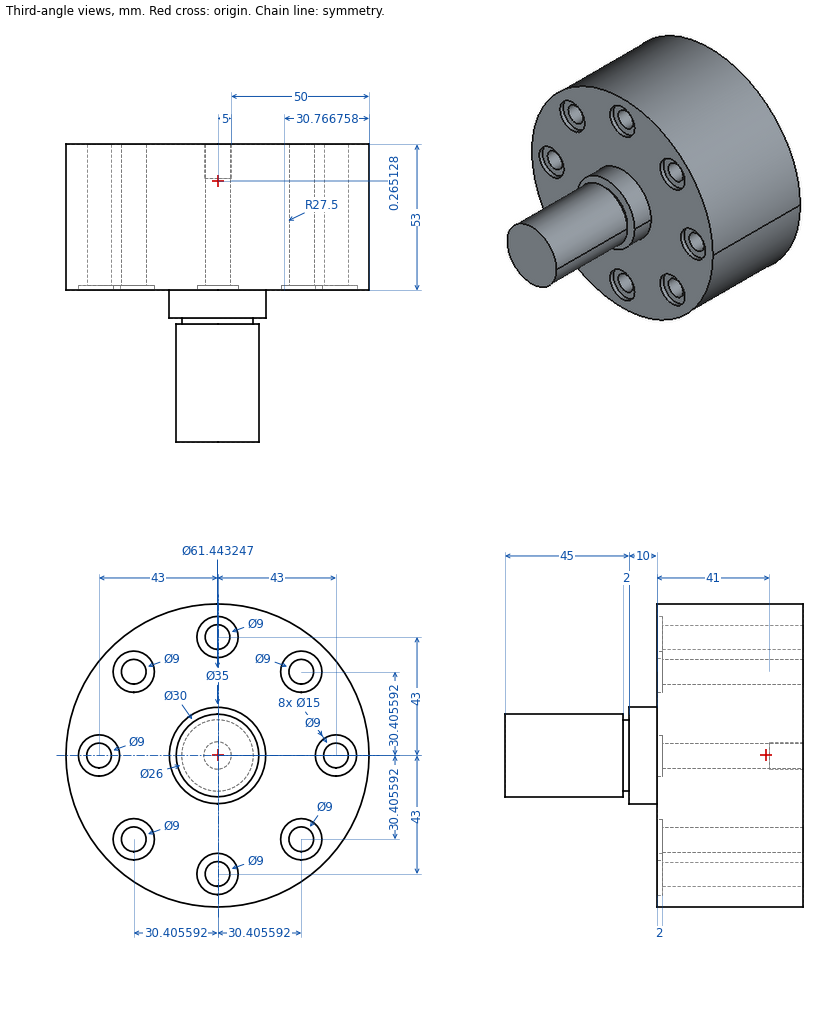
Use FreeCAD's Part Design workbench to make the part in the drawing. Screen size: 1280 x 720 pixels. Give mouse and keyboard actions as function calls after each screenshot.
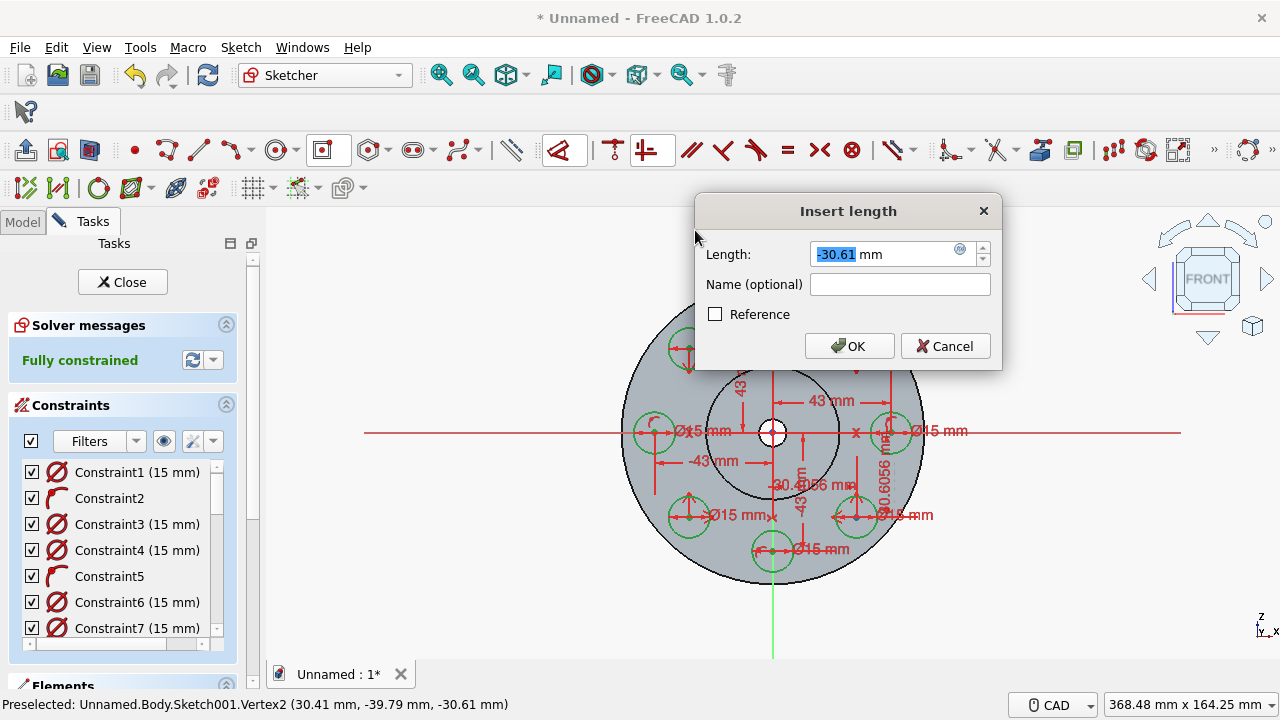
text(-30.405592)
key(Return)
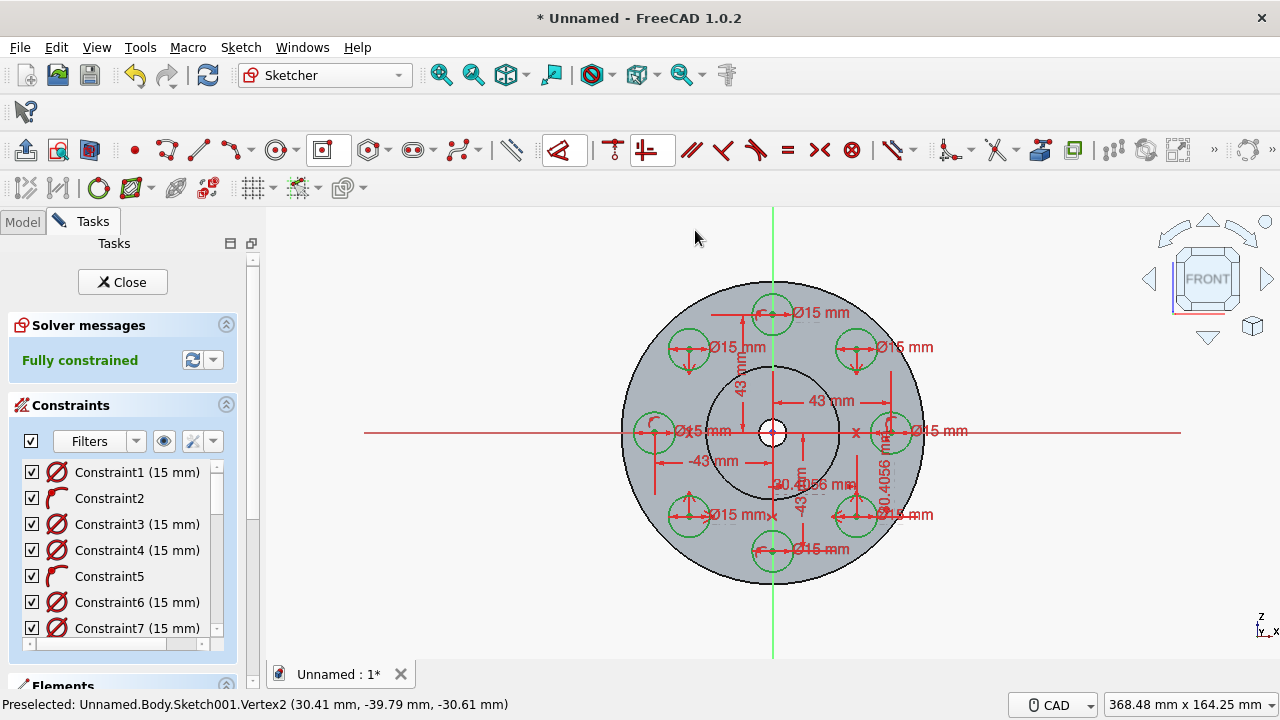
click(123, 282)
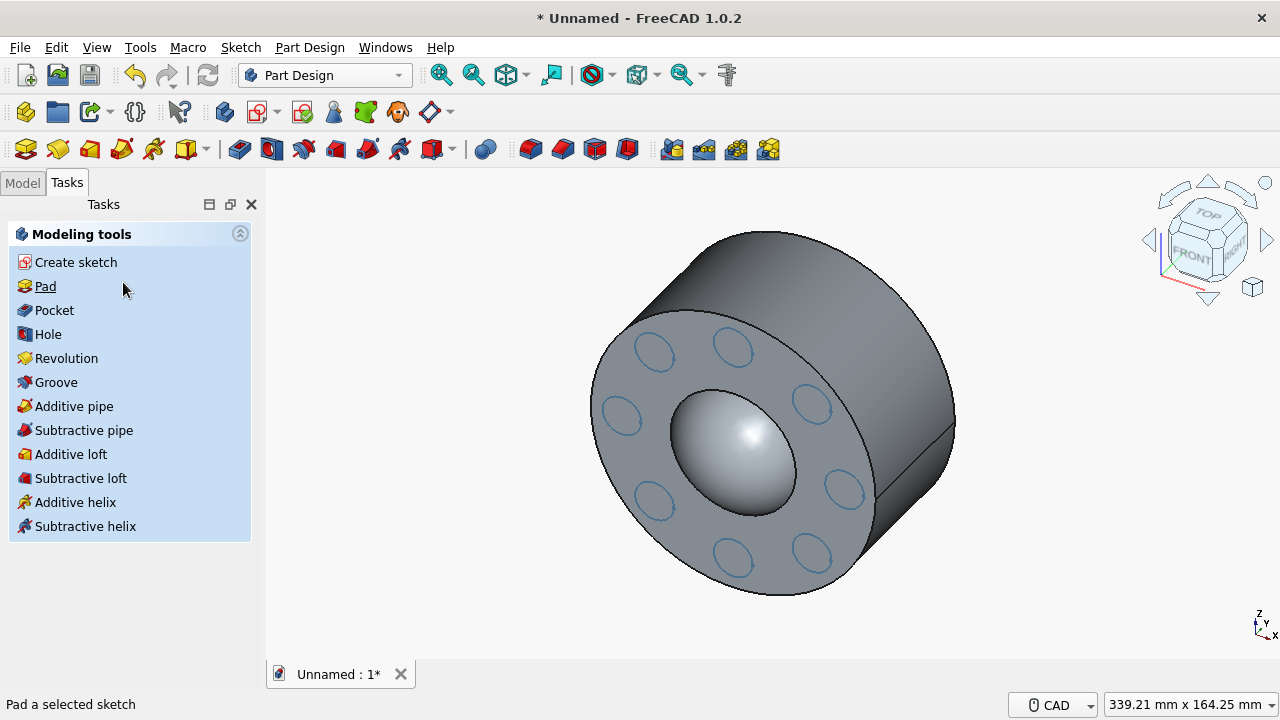
click(240, 150)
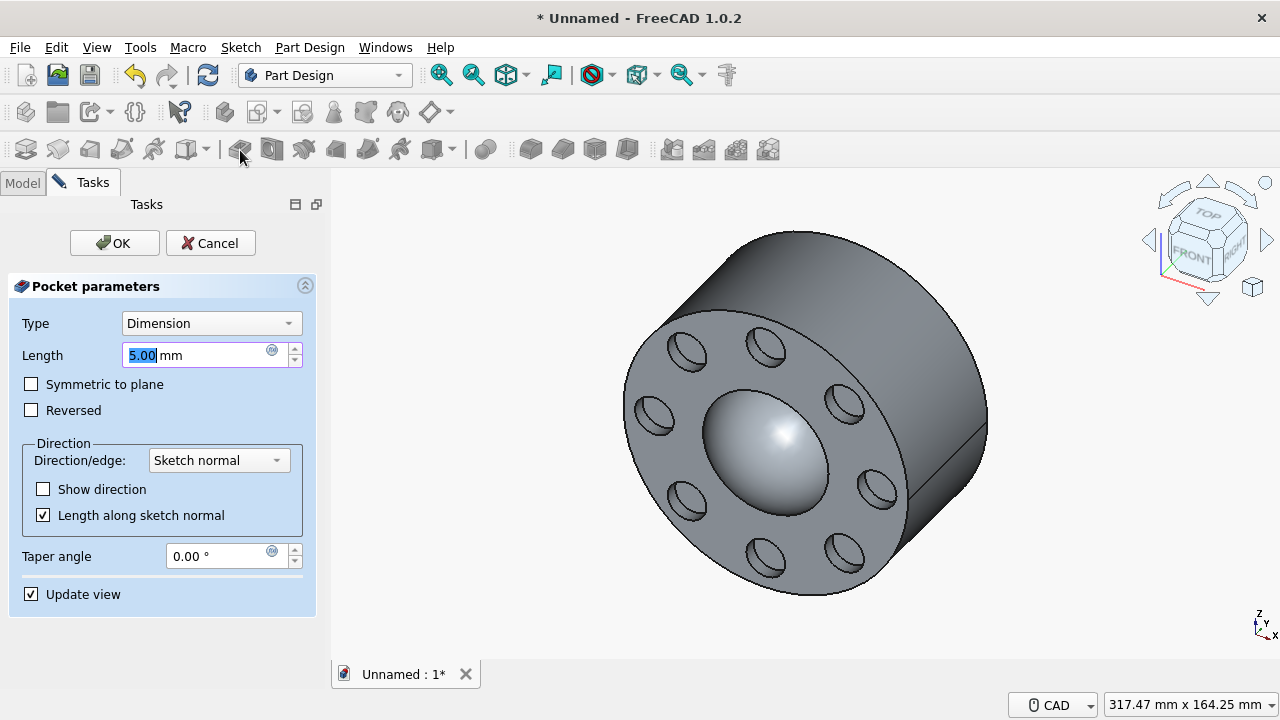
text(2)
key(Tab)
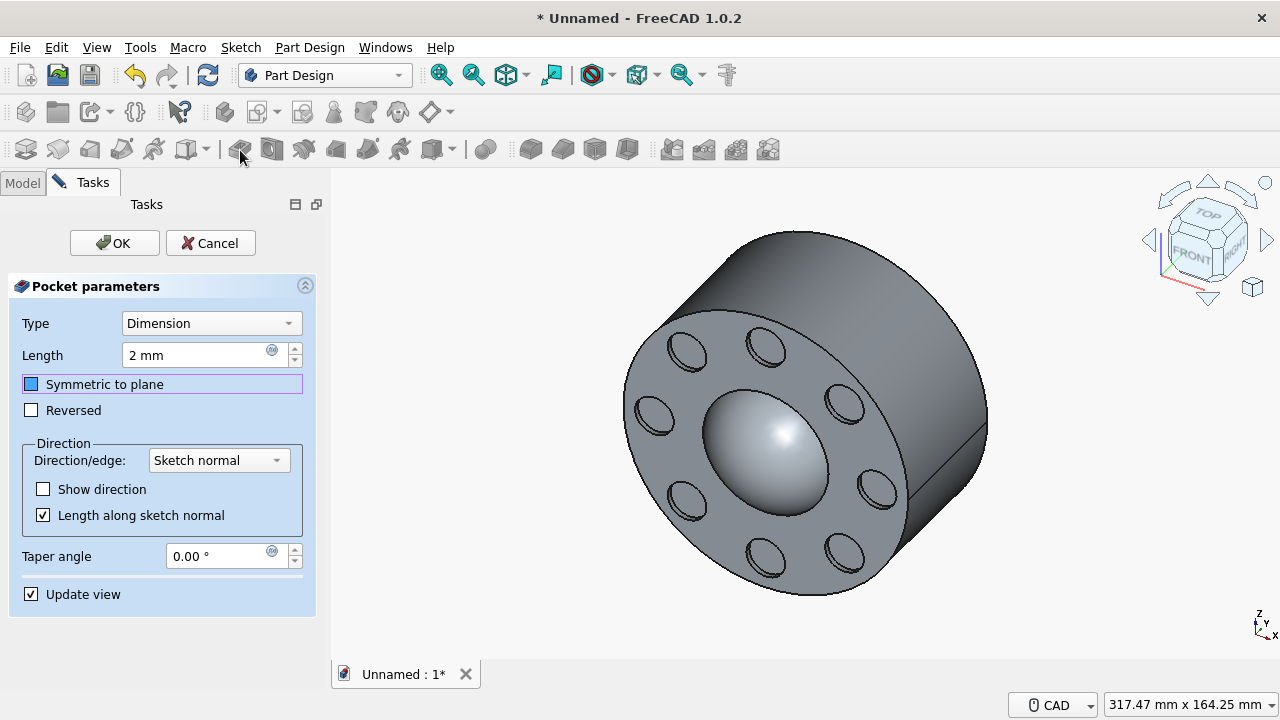
click(115, 243)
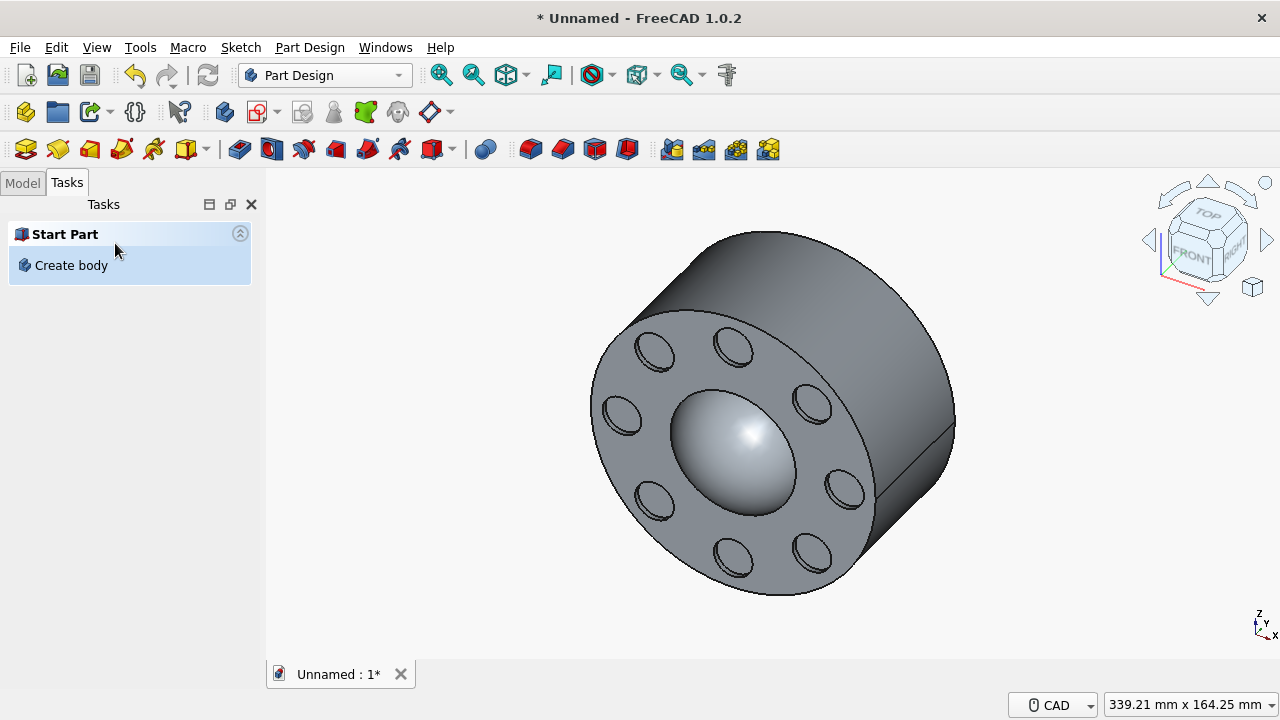
click(658, 348)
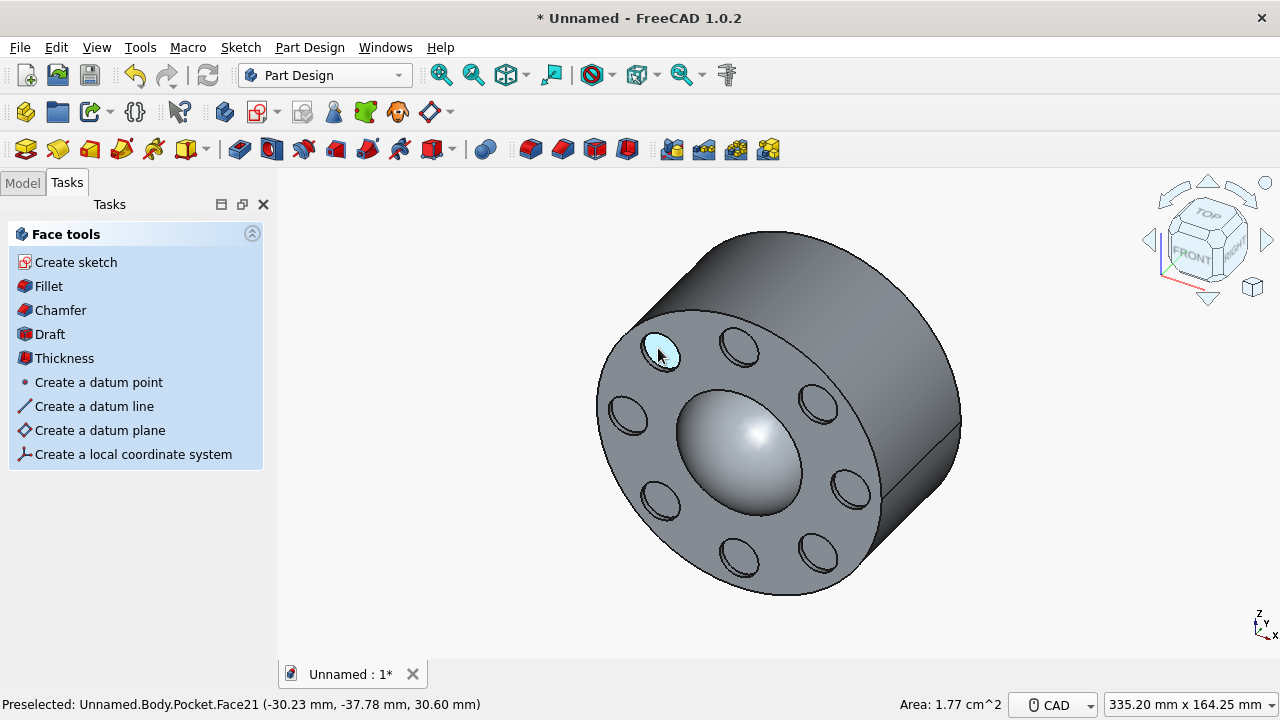
click(258, 112)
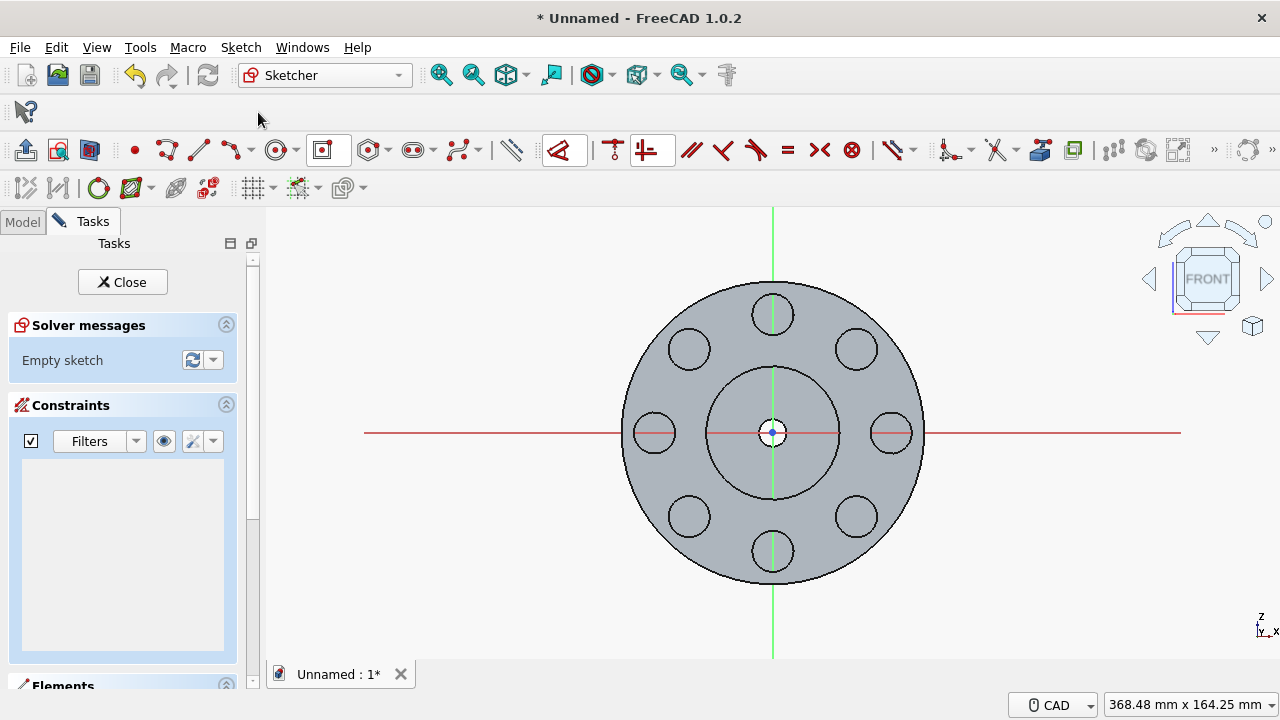
scroll(780, 303, up, 12)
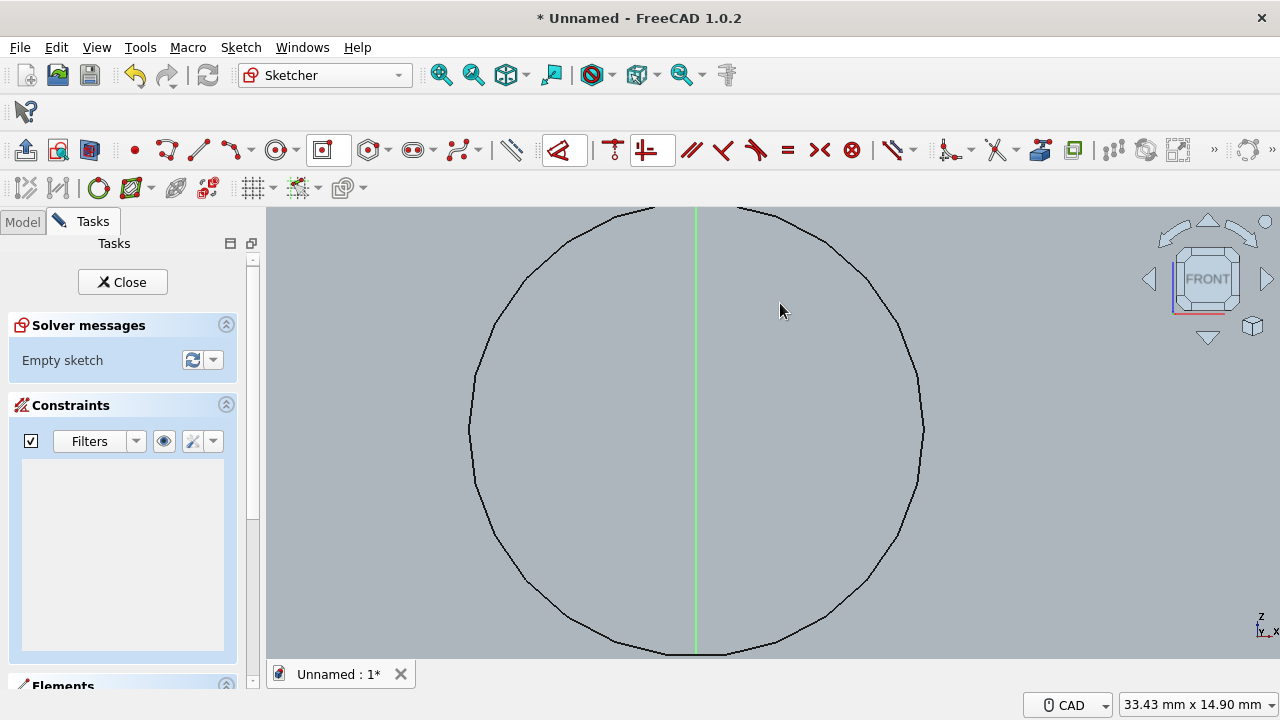
key(g)
key(c)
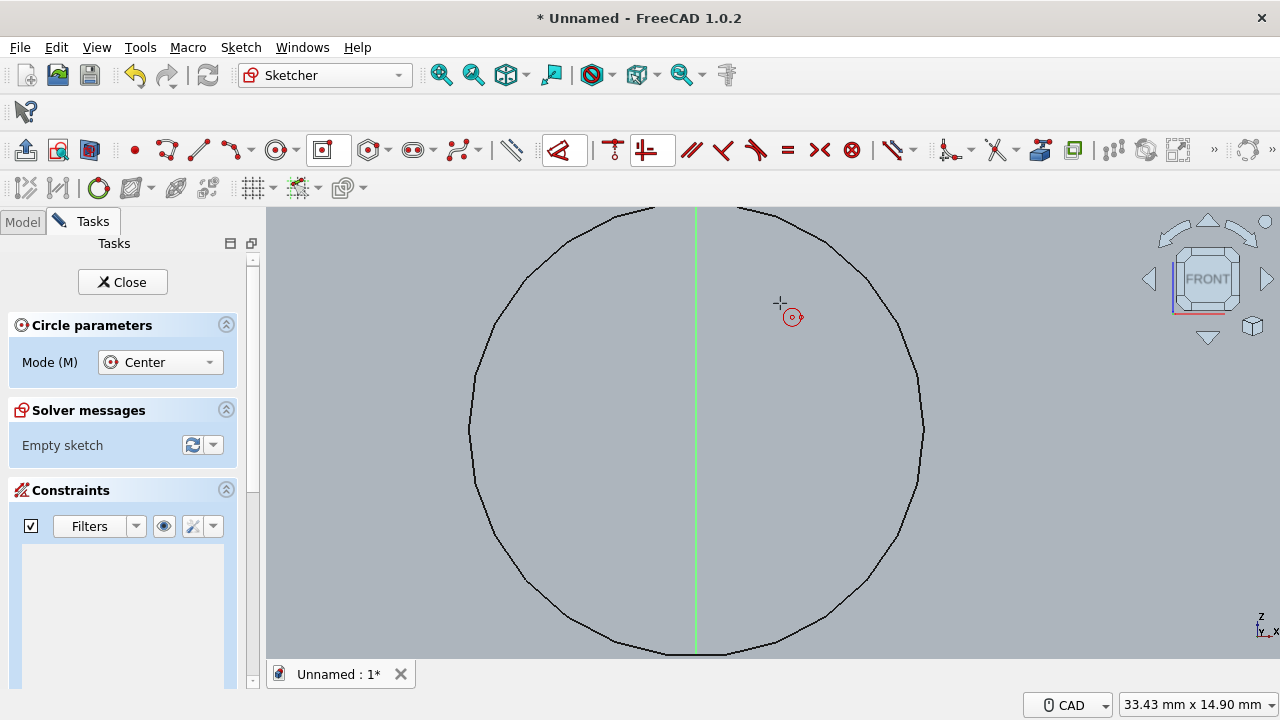
click(696, 430)
move(793, 333)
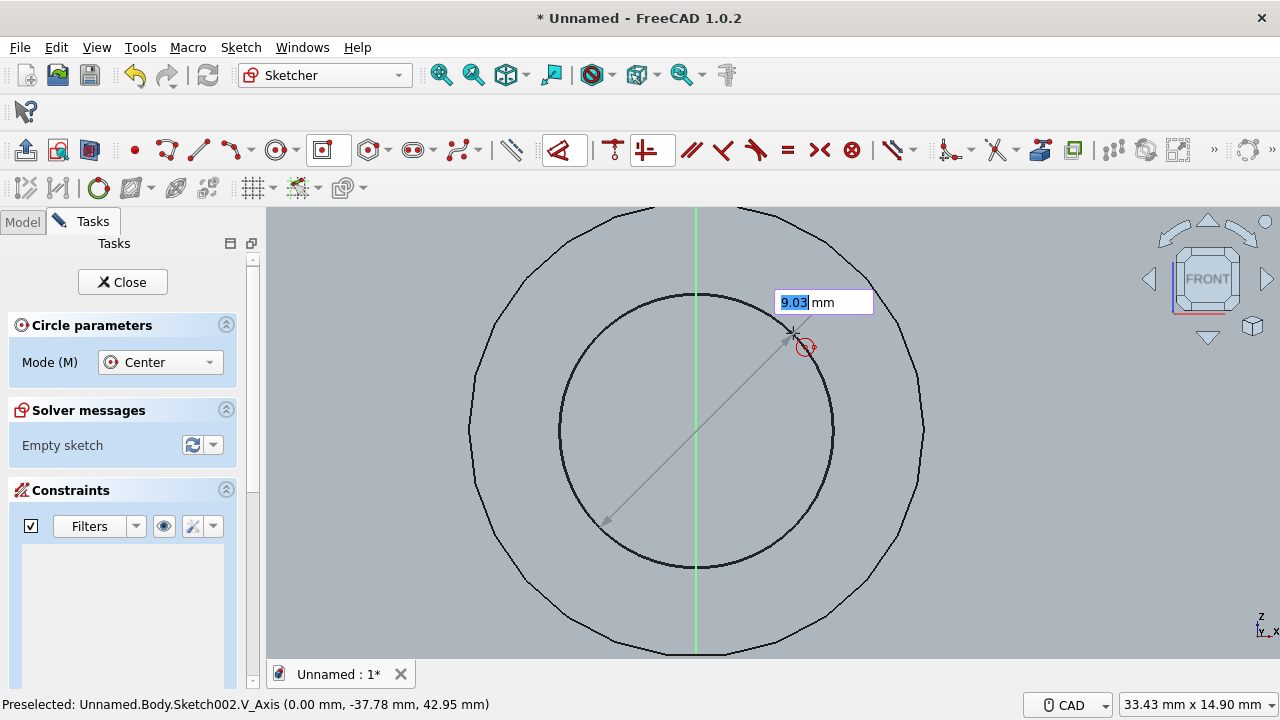
text(9)
key(Return)
key(Escape)